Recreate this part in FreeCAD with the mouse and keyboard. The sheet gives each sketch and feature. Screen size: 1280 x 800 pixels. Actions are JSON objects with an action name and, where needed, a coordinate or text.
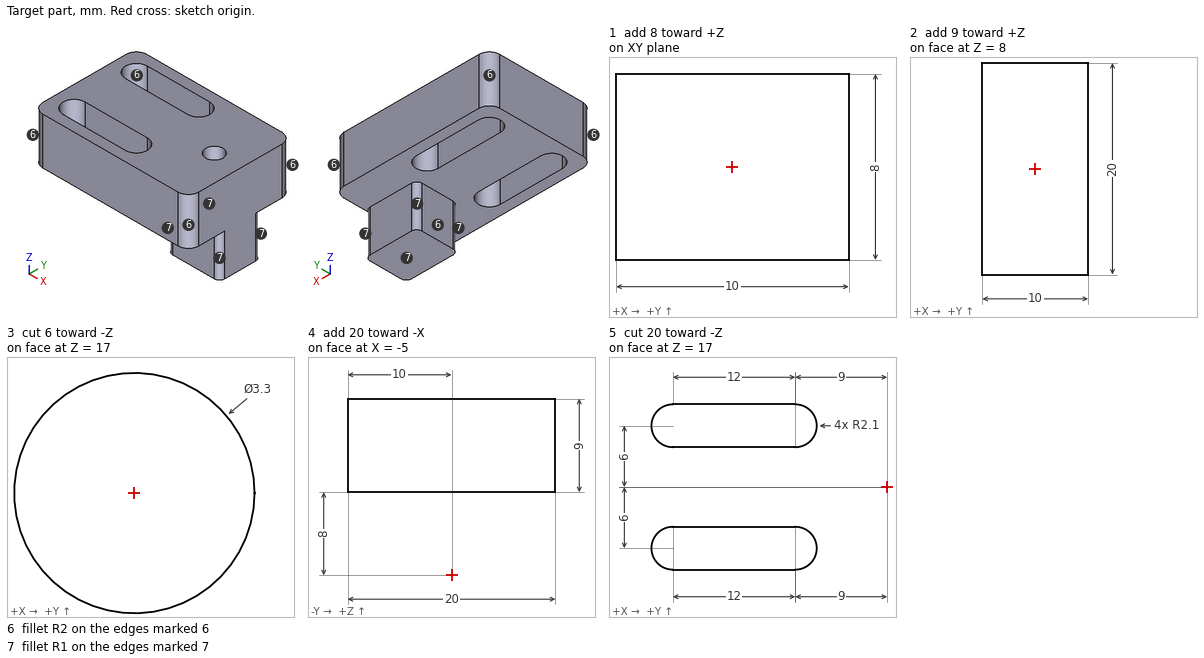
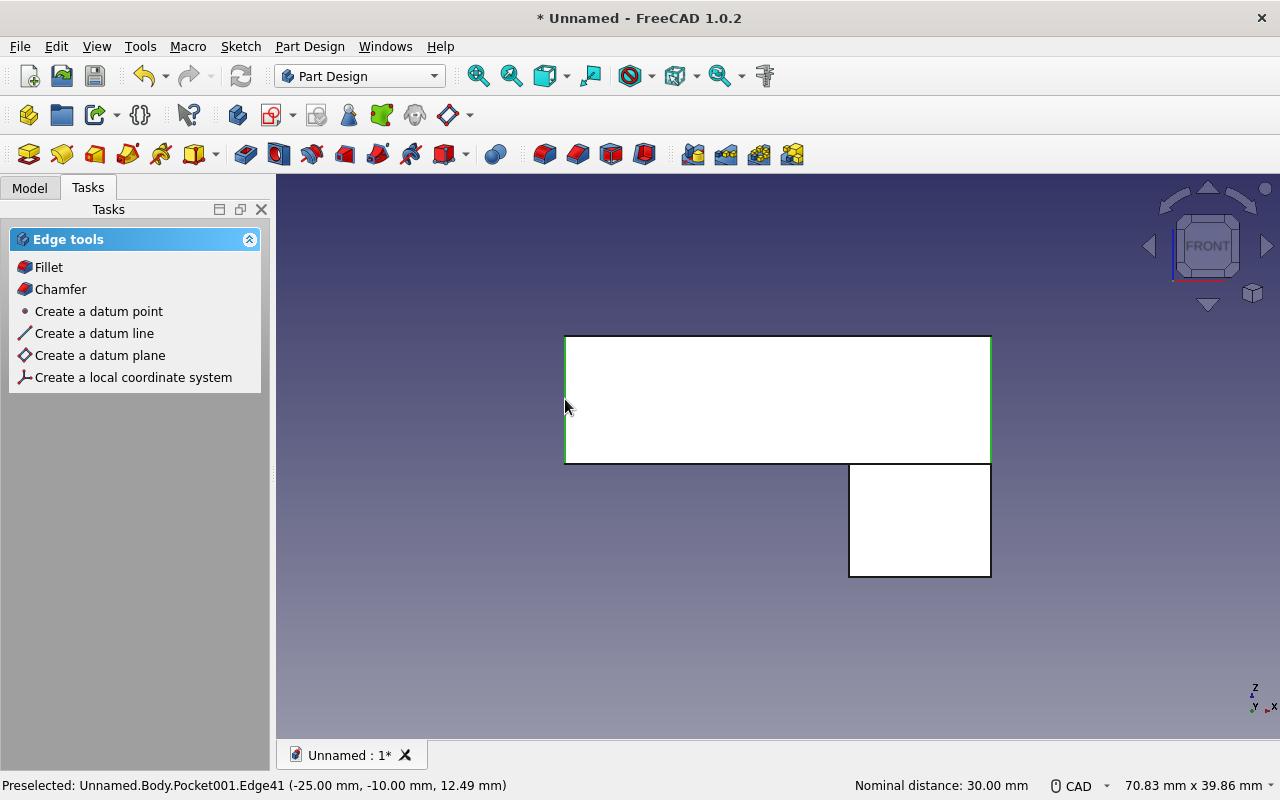
{"action": "key", "text": "3"}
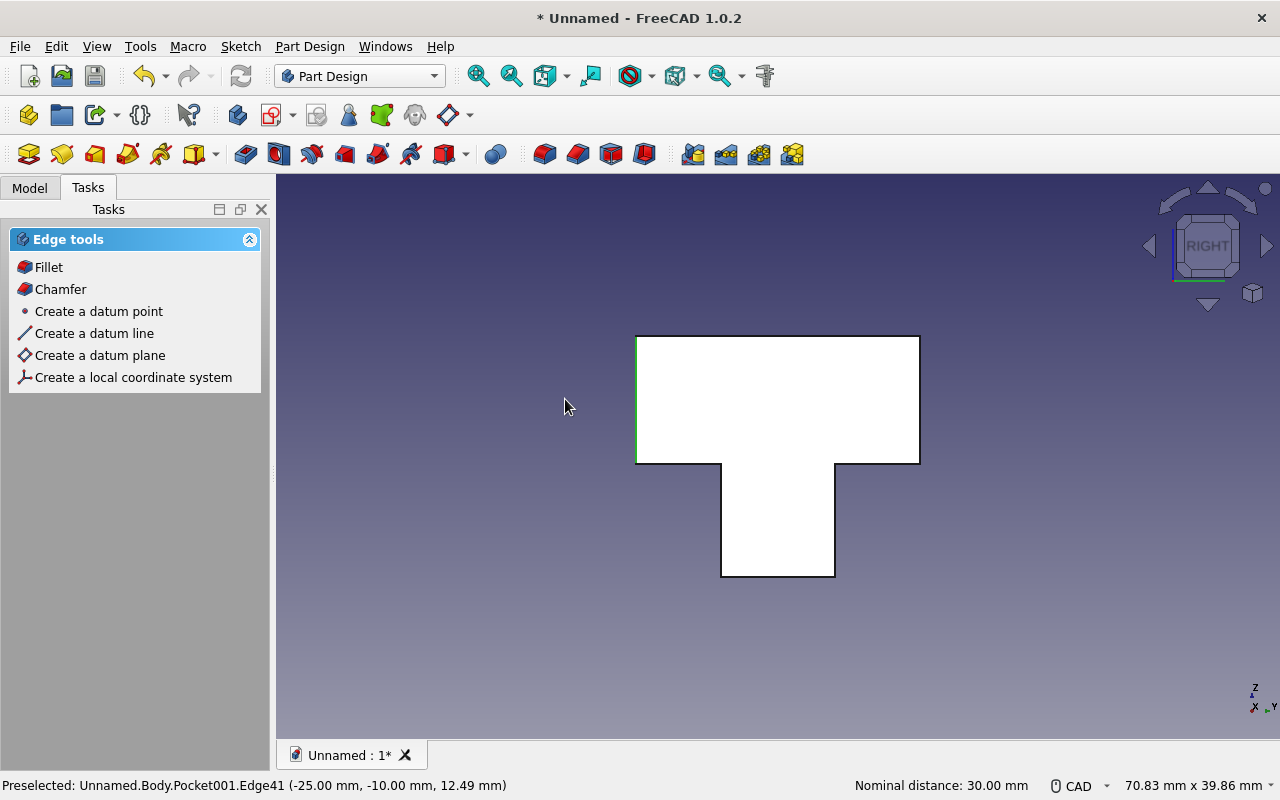
{"action": "left_click", "coordinate": [479, 76]}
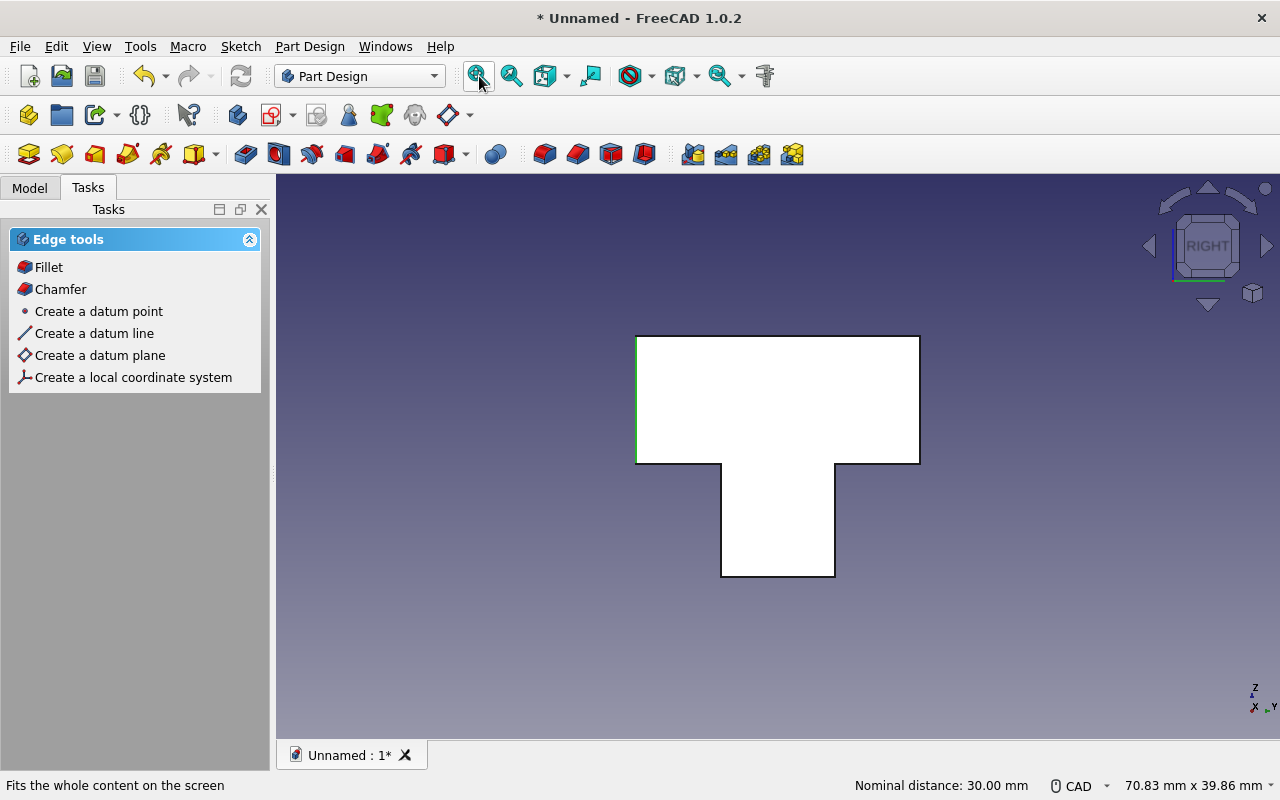
{"action": "left_click", "coordinate": [920, 399], "text": "ctrl"}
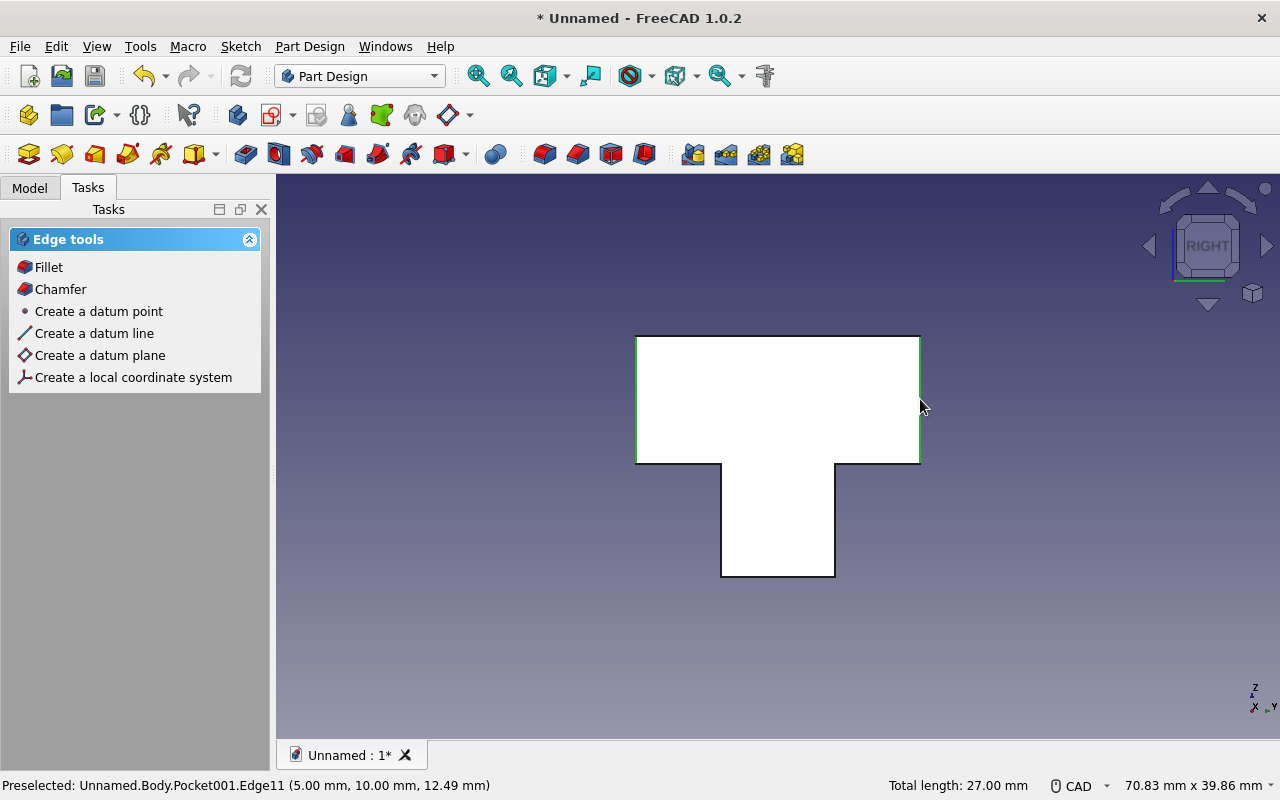
{"action": "key", "text": "5"}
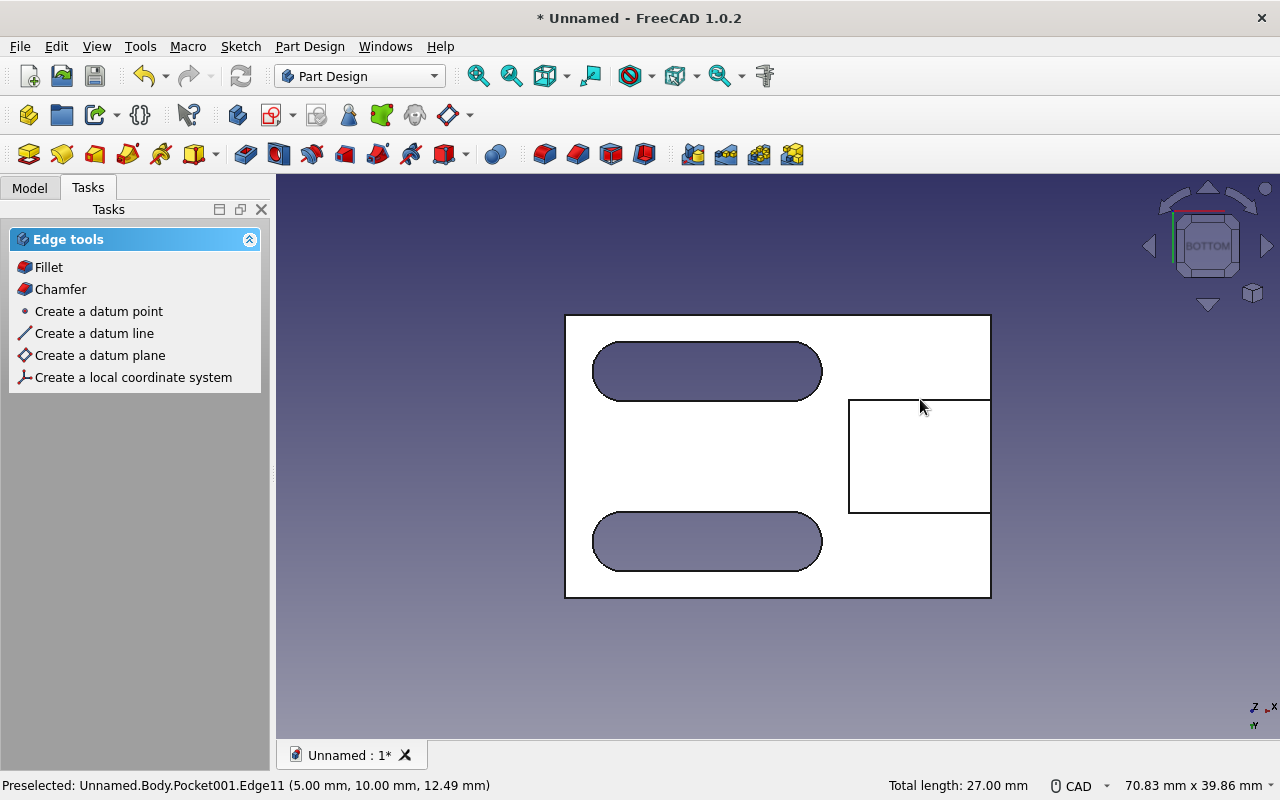
{"action": "key", "text": "4"}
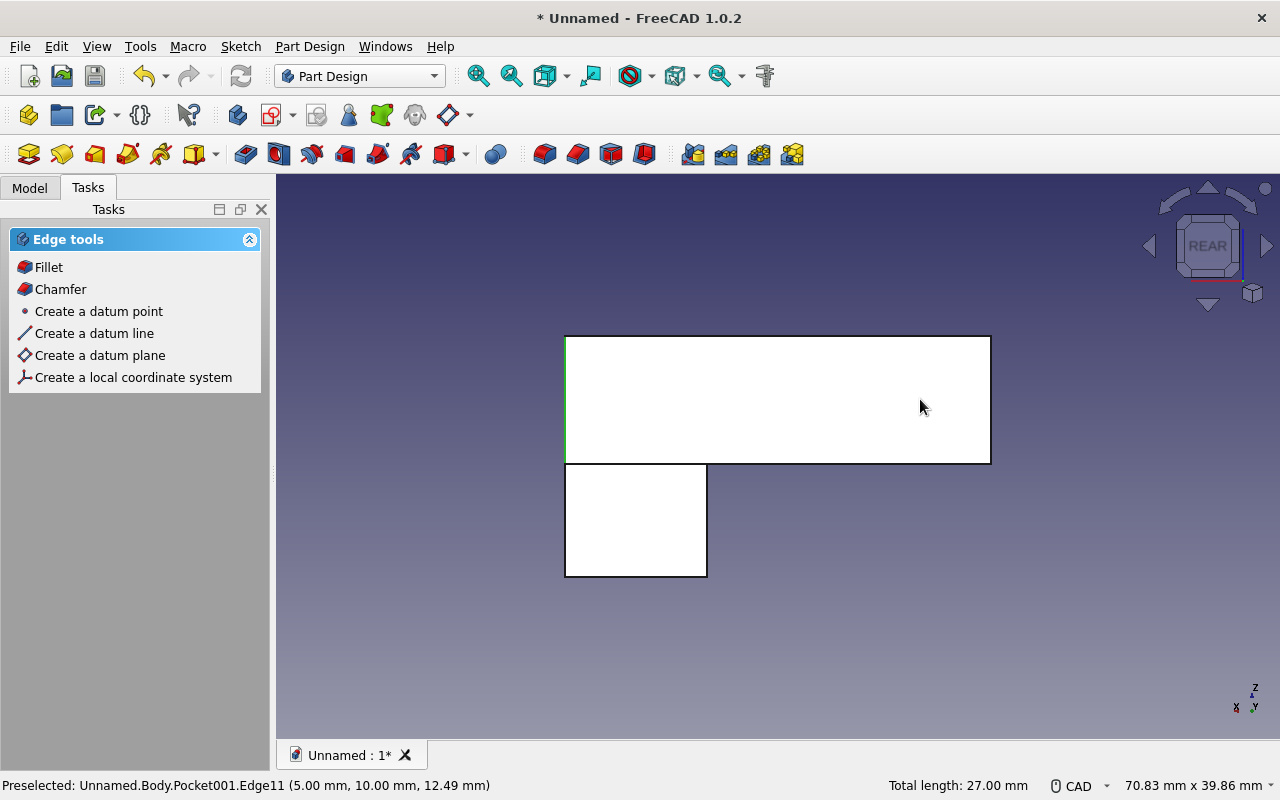
{"action": "key", "text": "v f"}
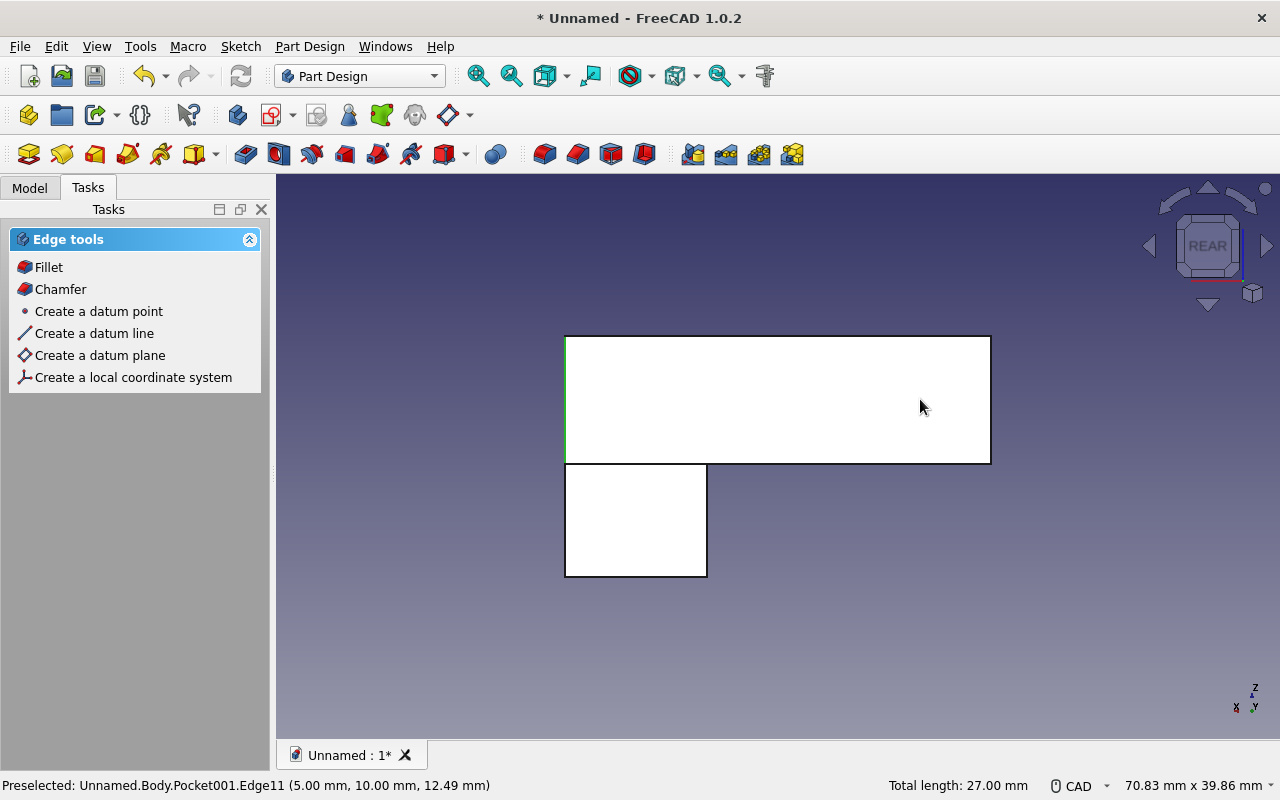
{"action": "left_click", "coordinate": [991, 399], "text": "ctrl"}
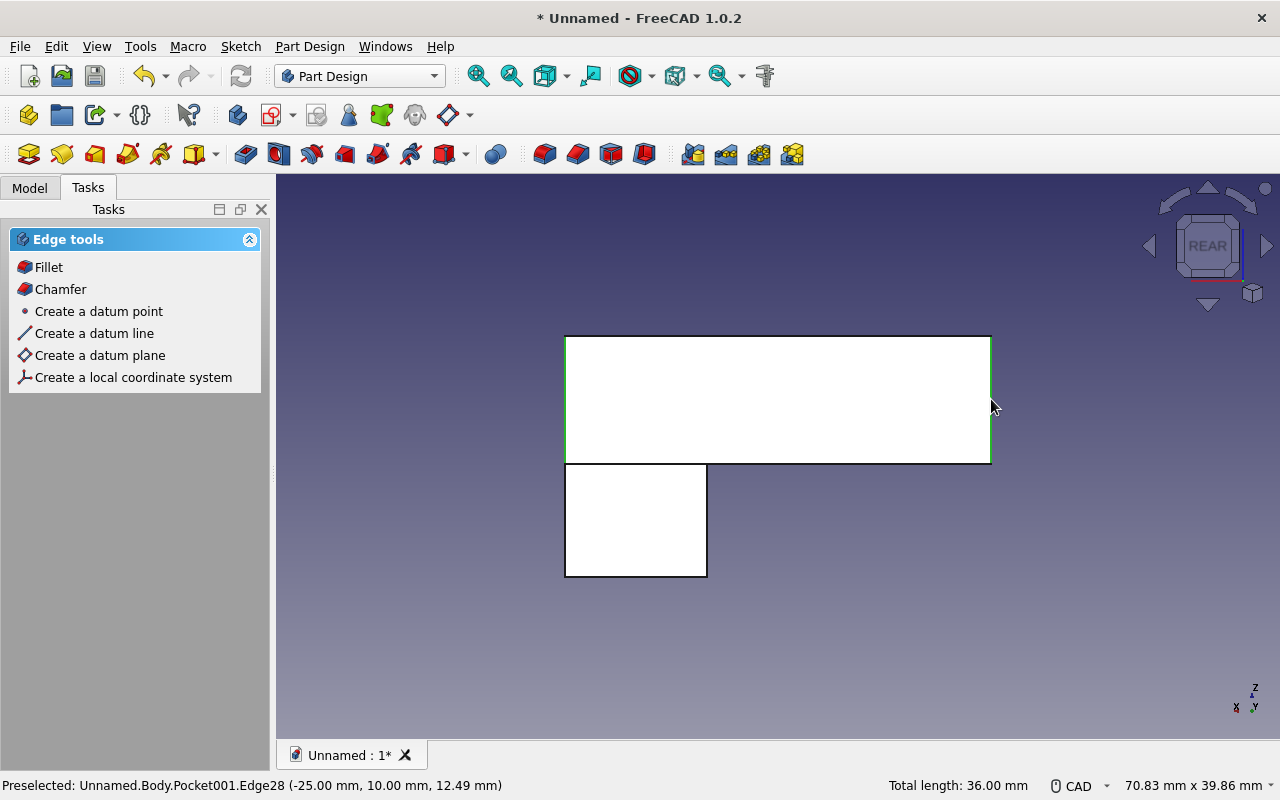
{"action": "left_click", "coordinate": [545, 154]}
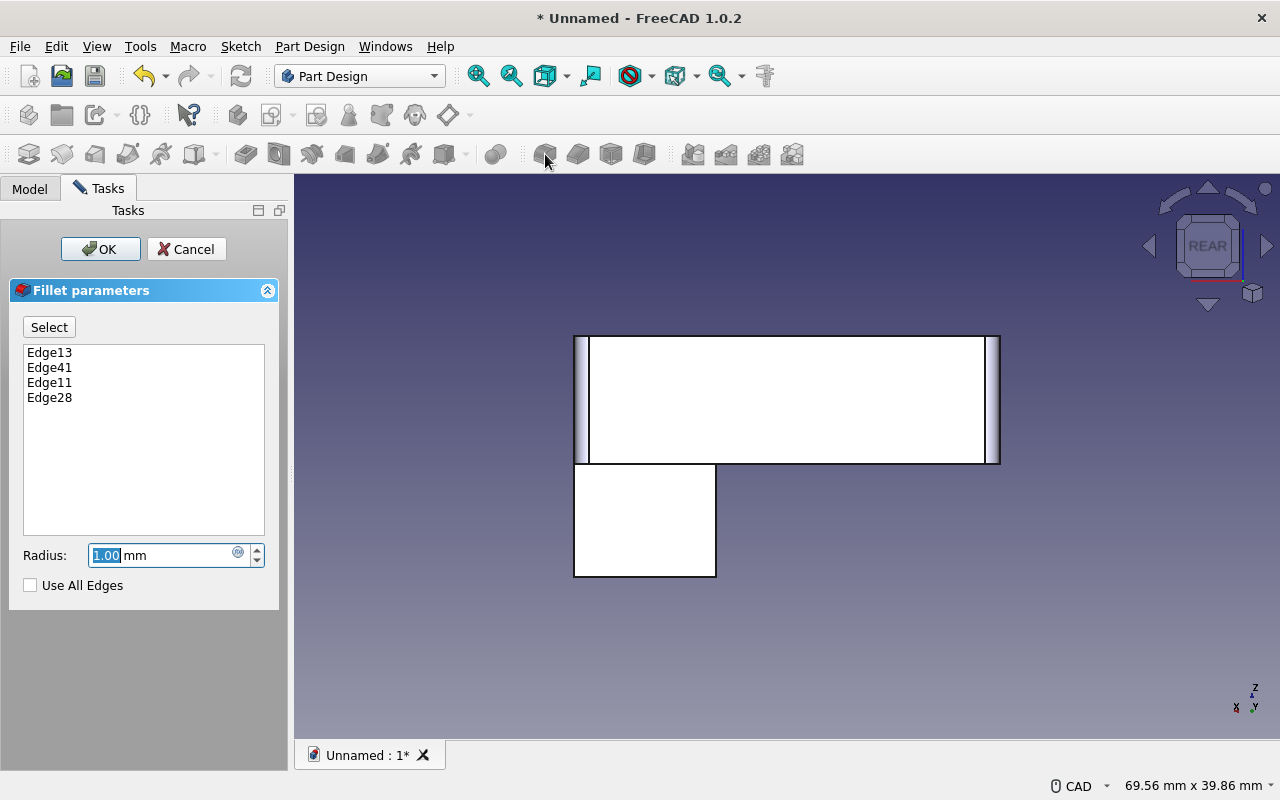
{"action": "type", "text": "2"}
{"action": "key", "text": "Tab"}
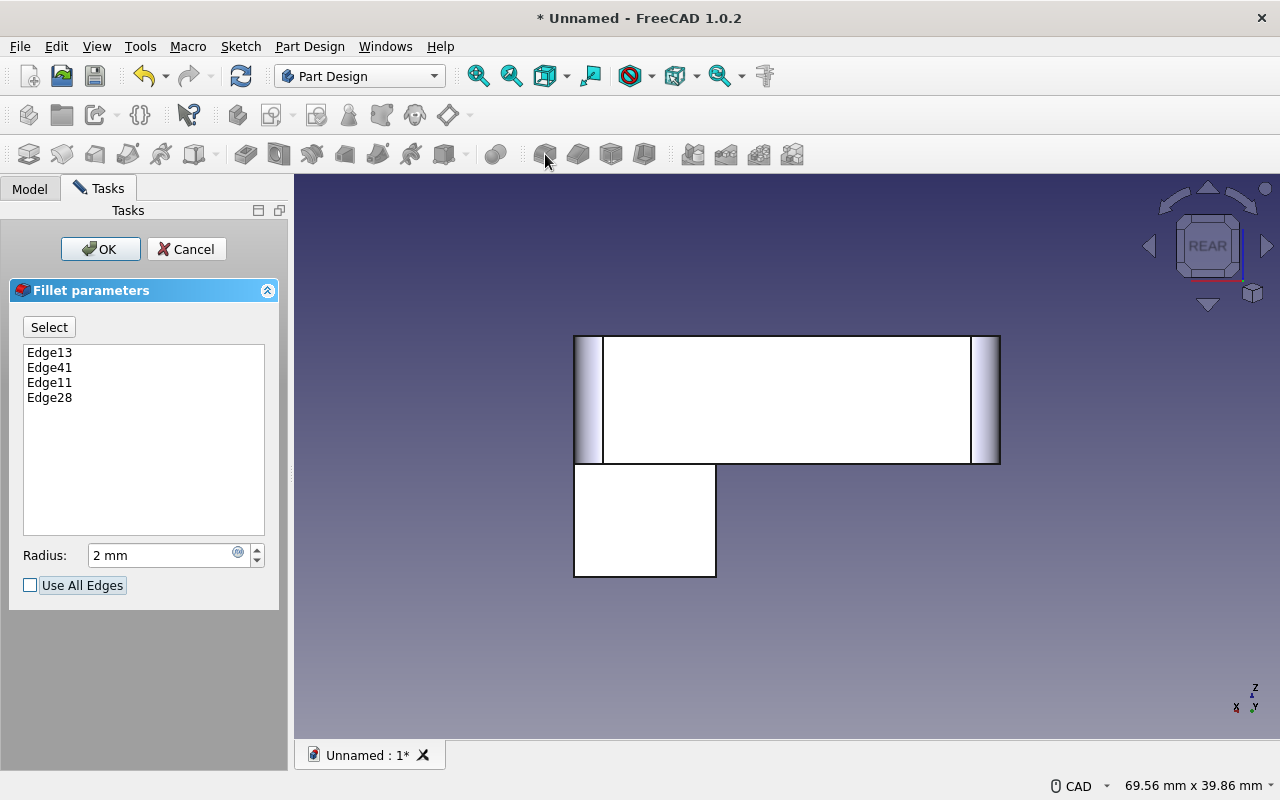
{"action": "left_click", "coordinate": [101, 249]}